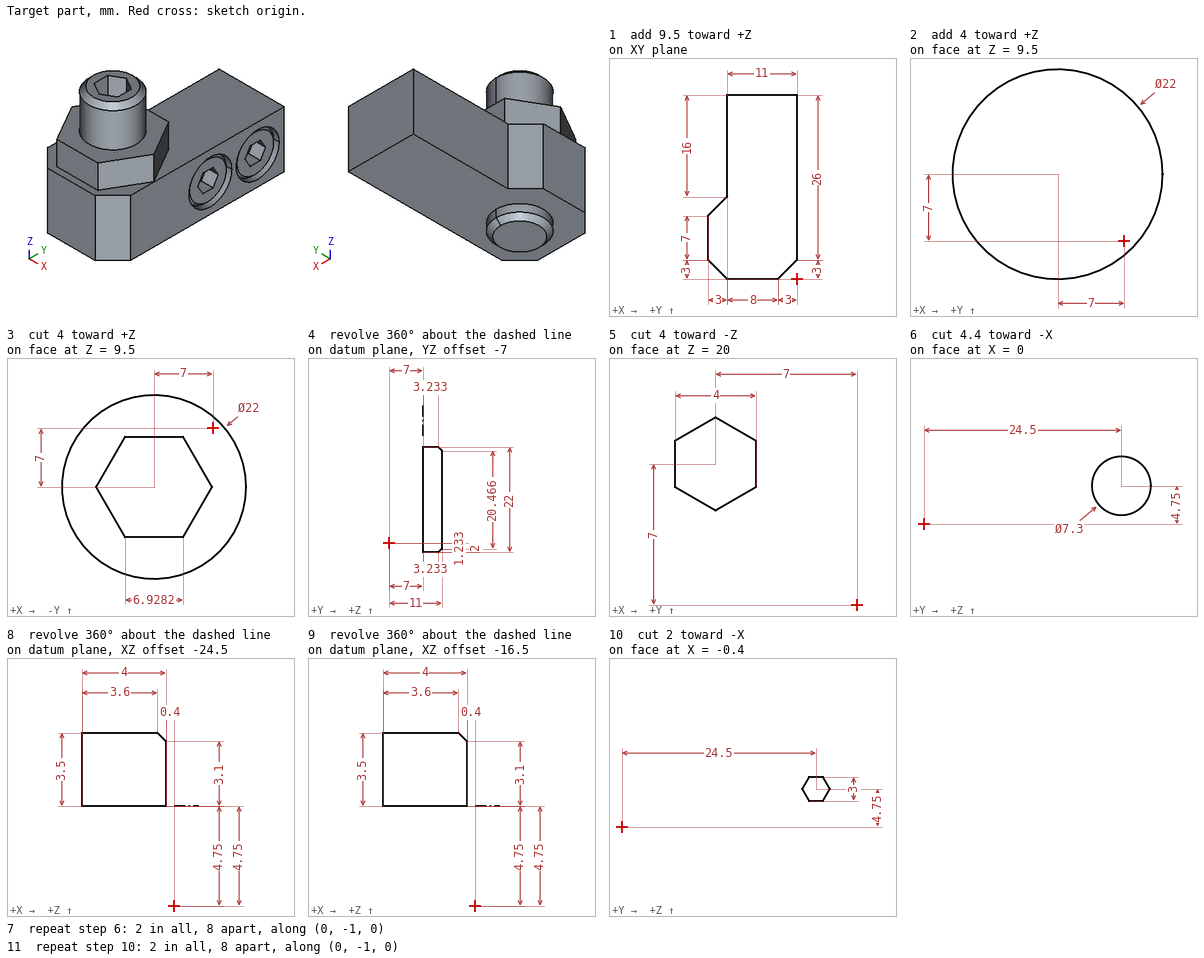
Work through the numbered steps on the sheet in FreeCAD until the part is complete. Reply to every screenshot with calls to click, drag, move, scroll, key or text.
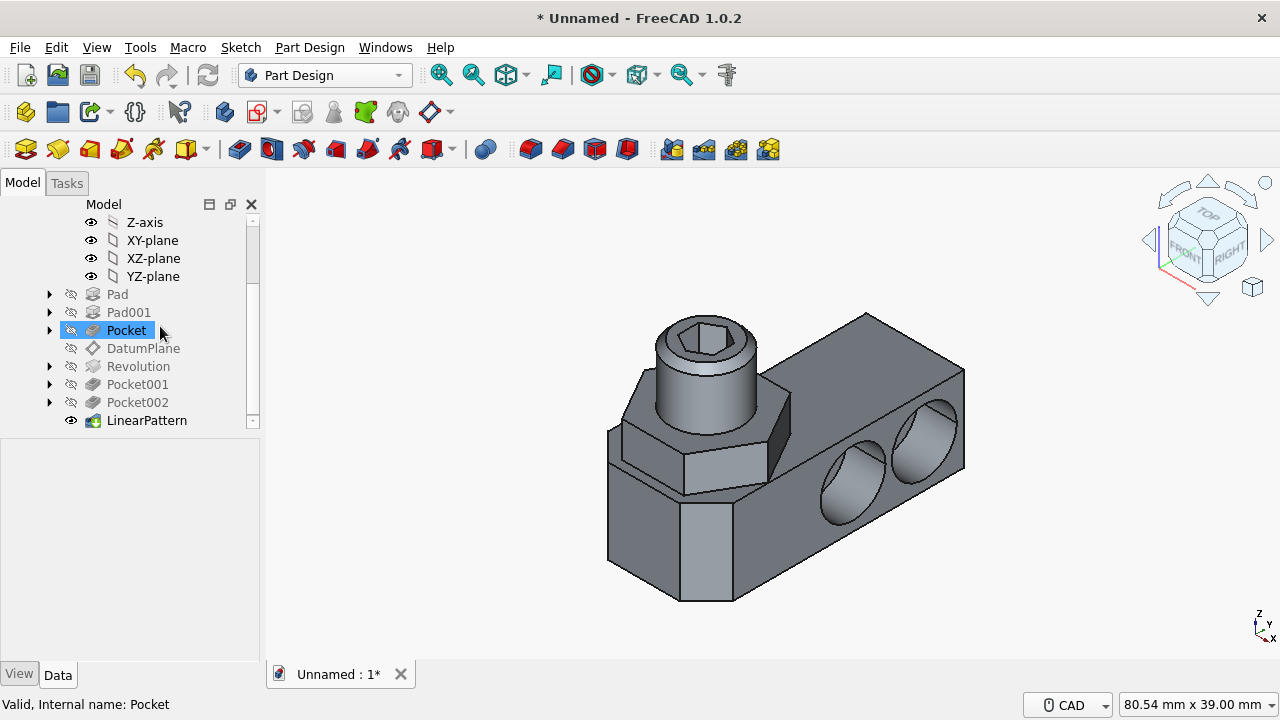
scroll(160, 326, up, 15)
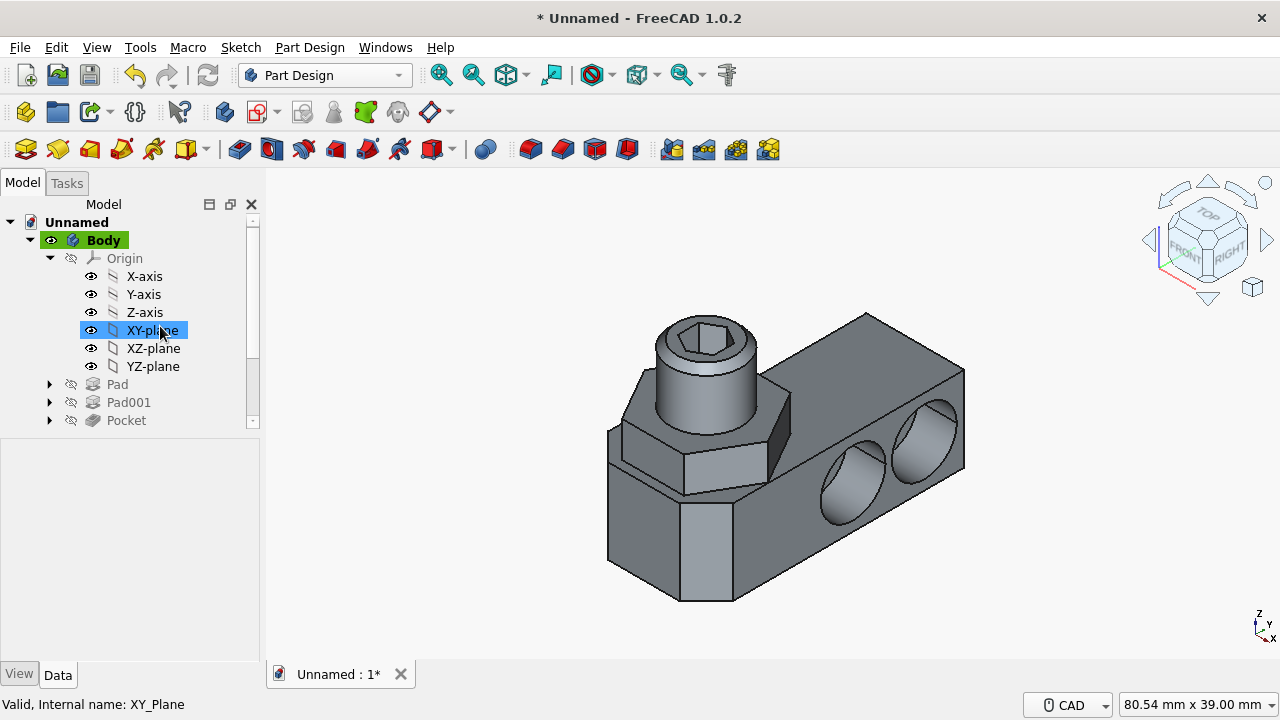
click(136, 348)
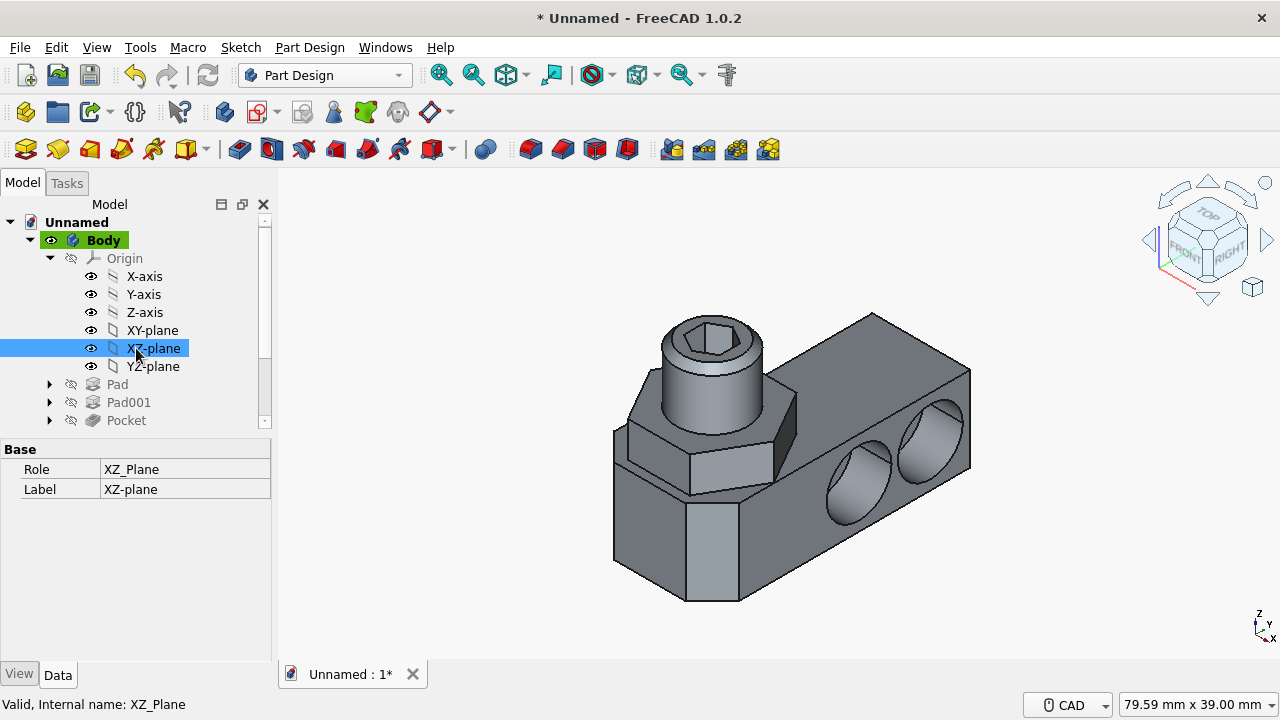
click(430, 112)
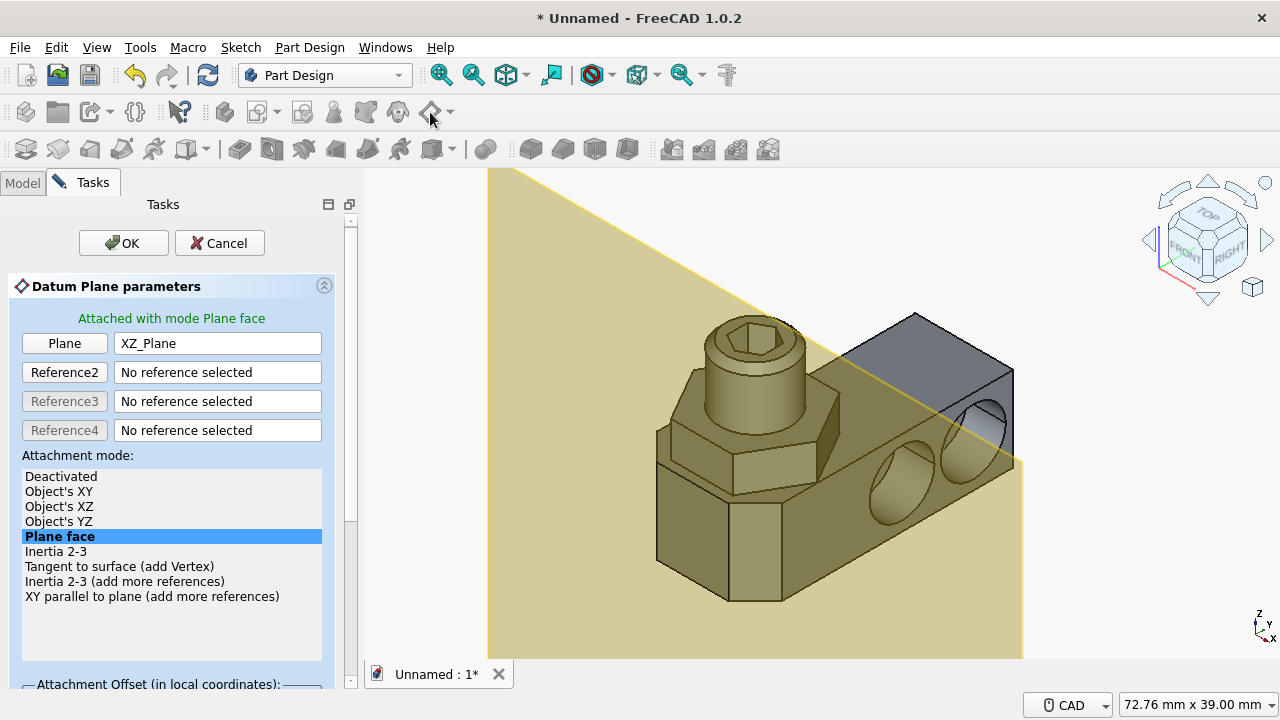
scroll(351, 451, down, 3)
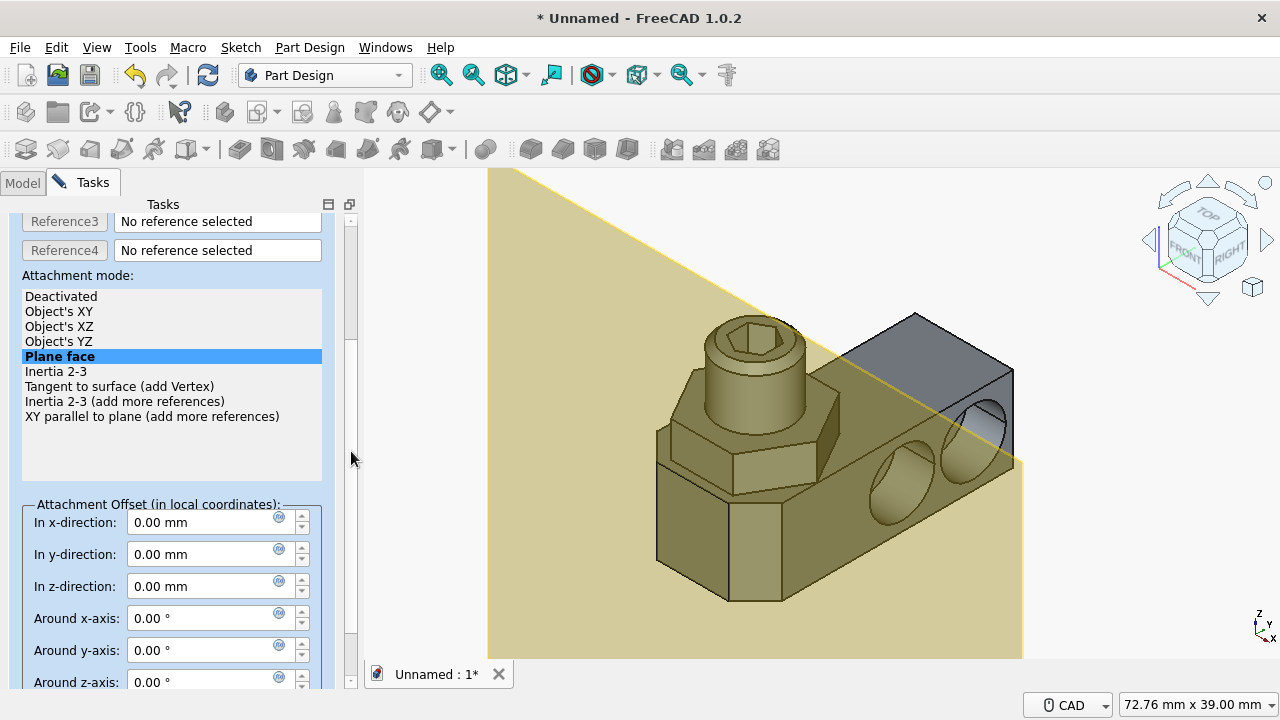
triple_click(210, 586)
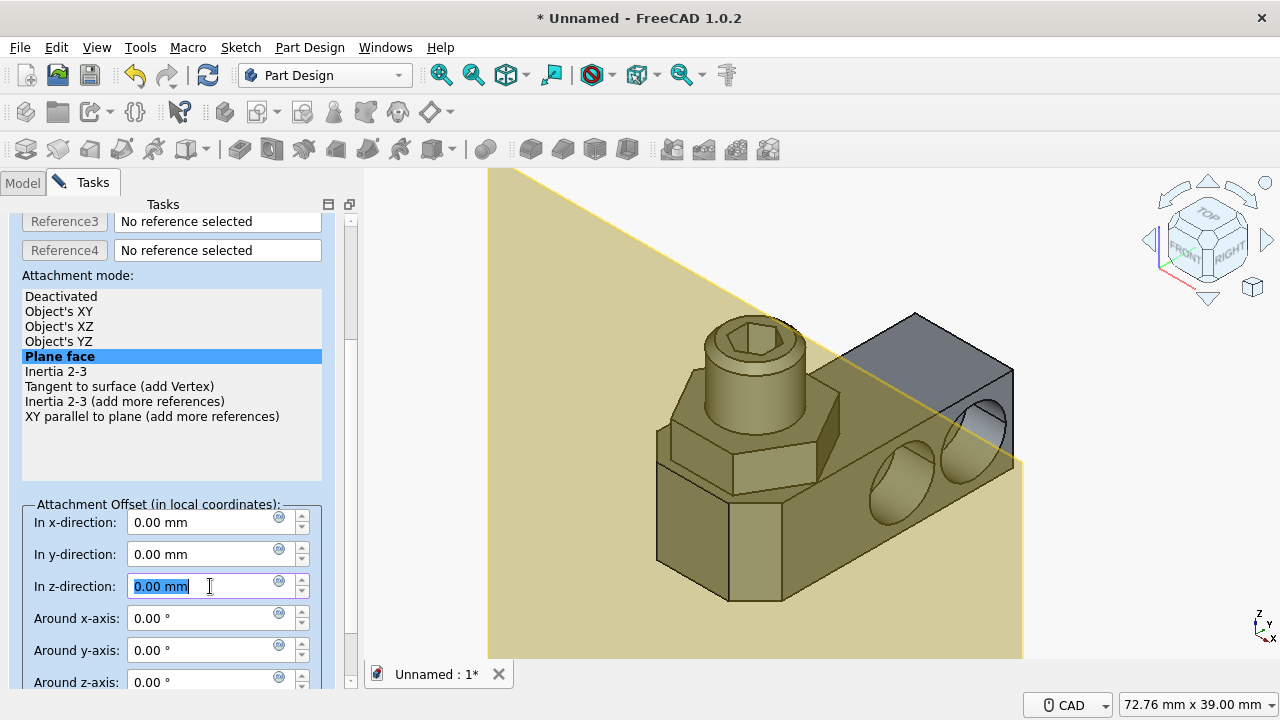
text(-24.5)
key(Tab)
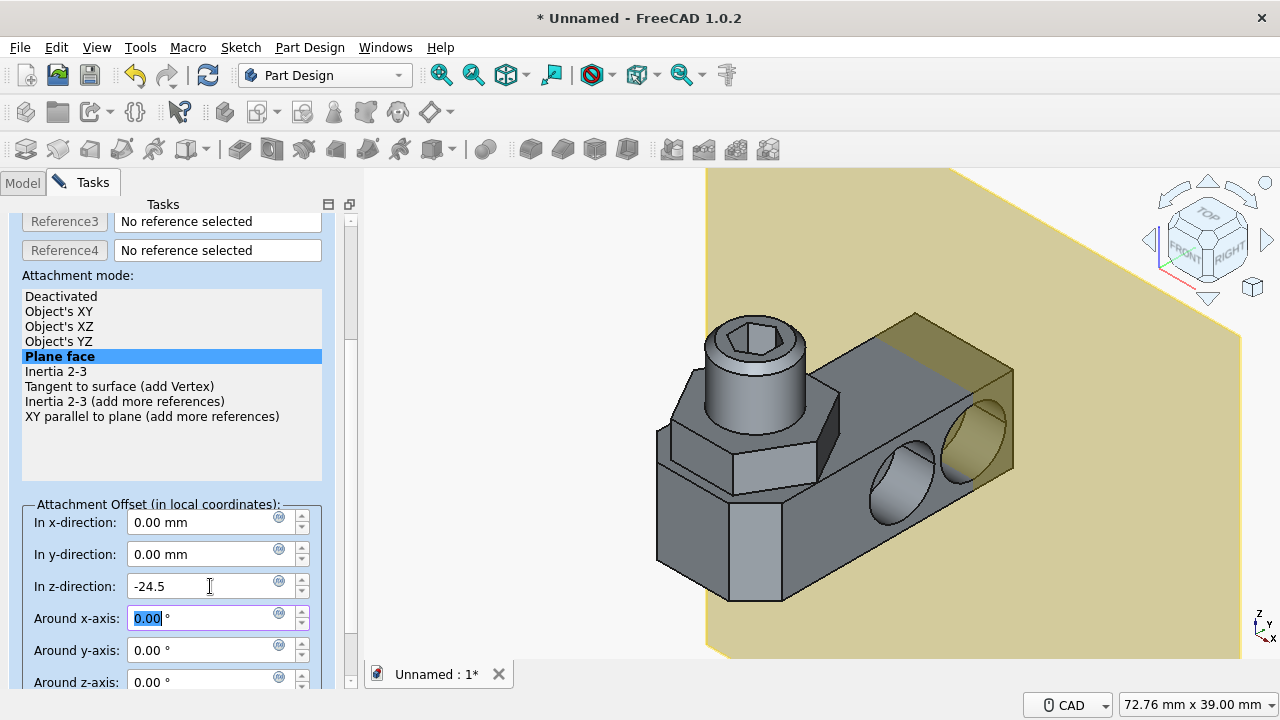
scroll(351, 451, up, 4)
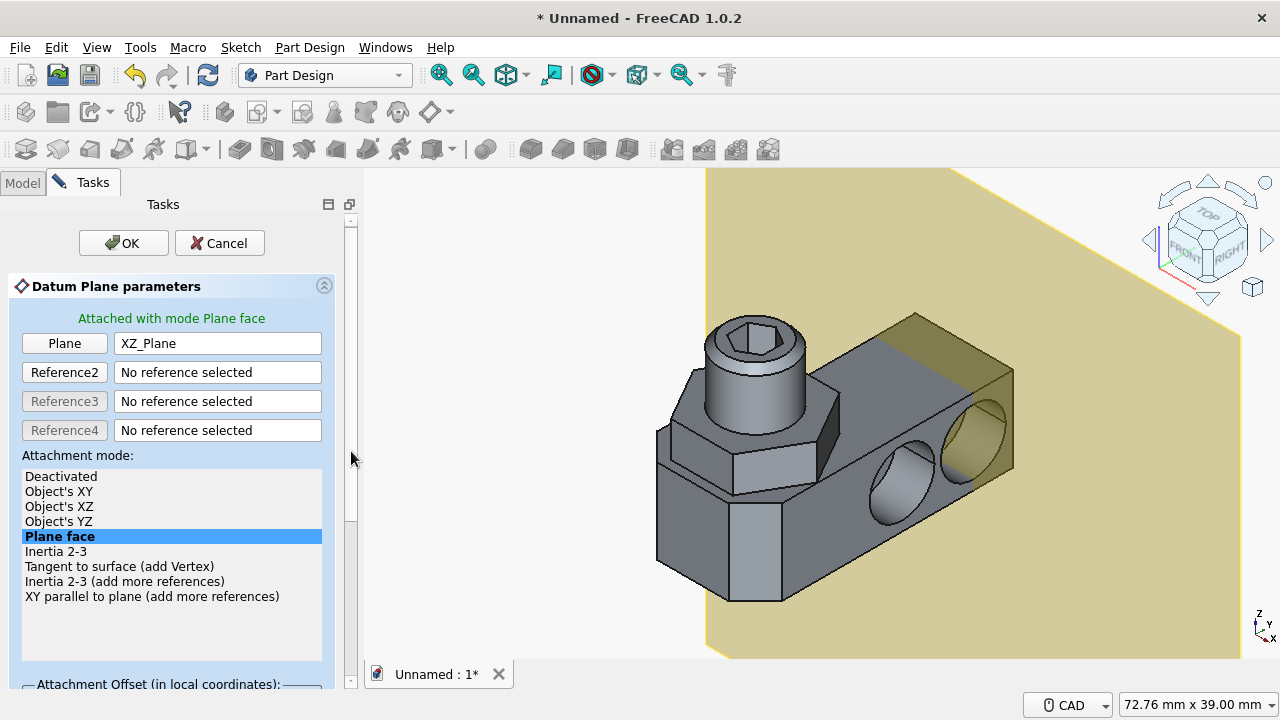
click(124, 243)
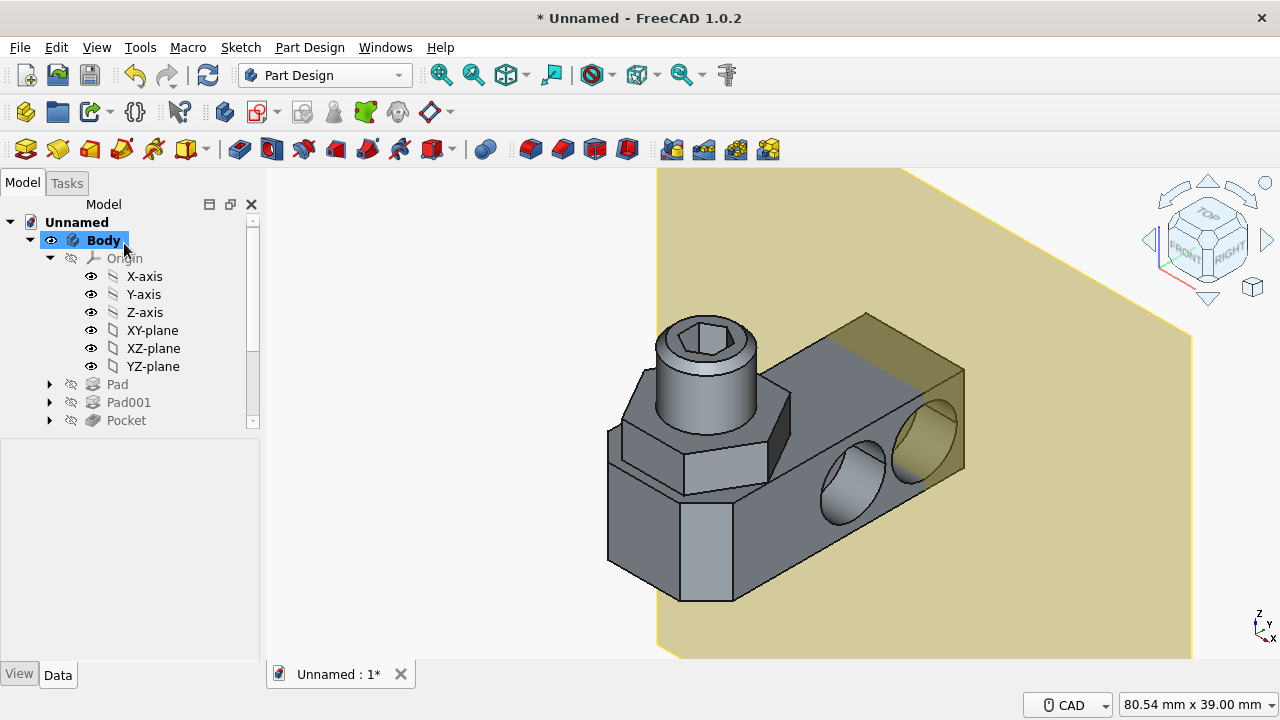
scroll(100, 326, down, 3)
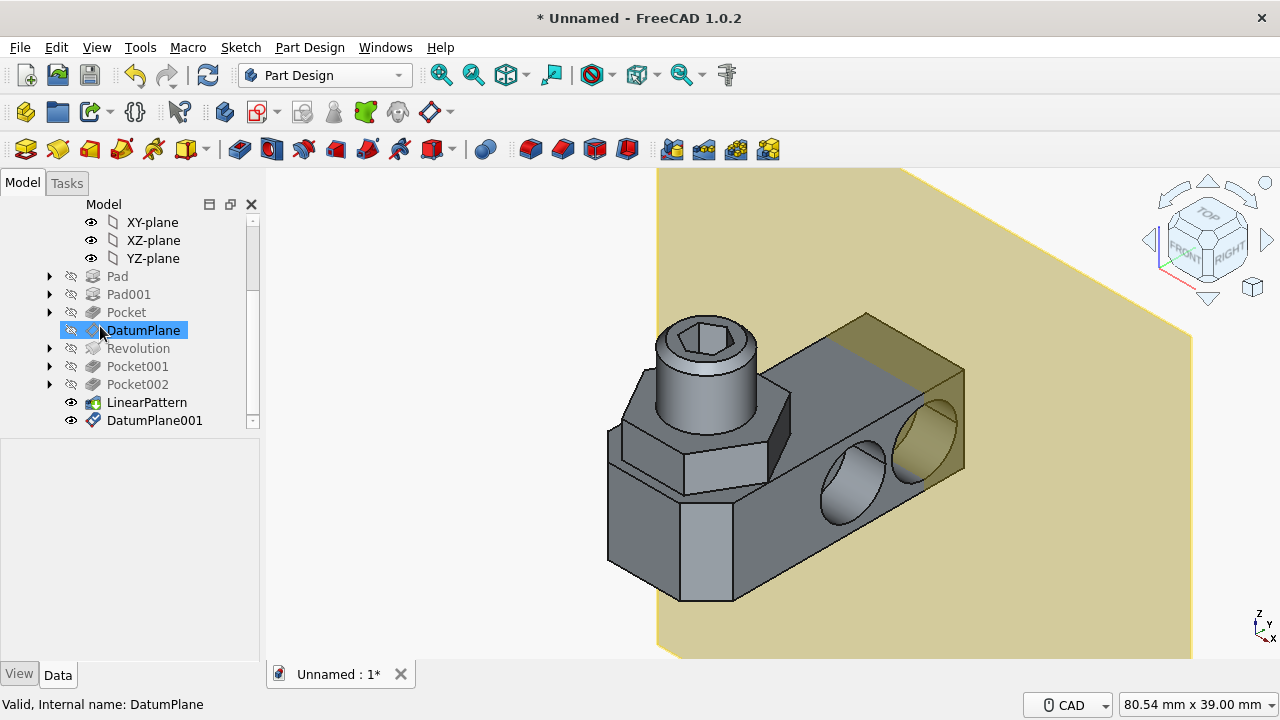
click(116, 420)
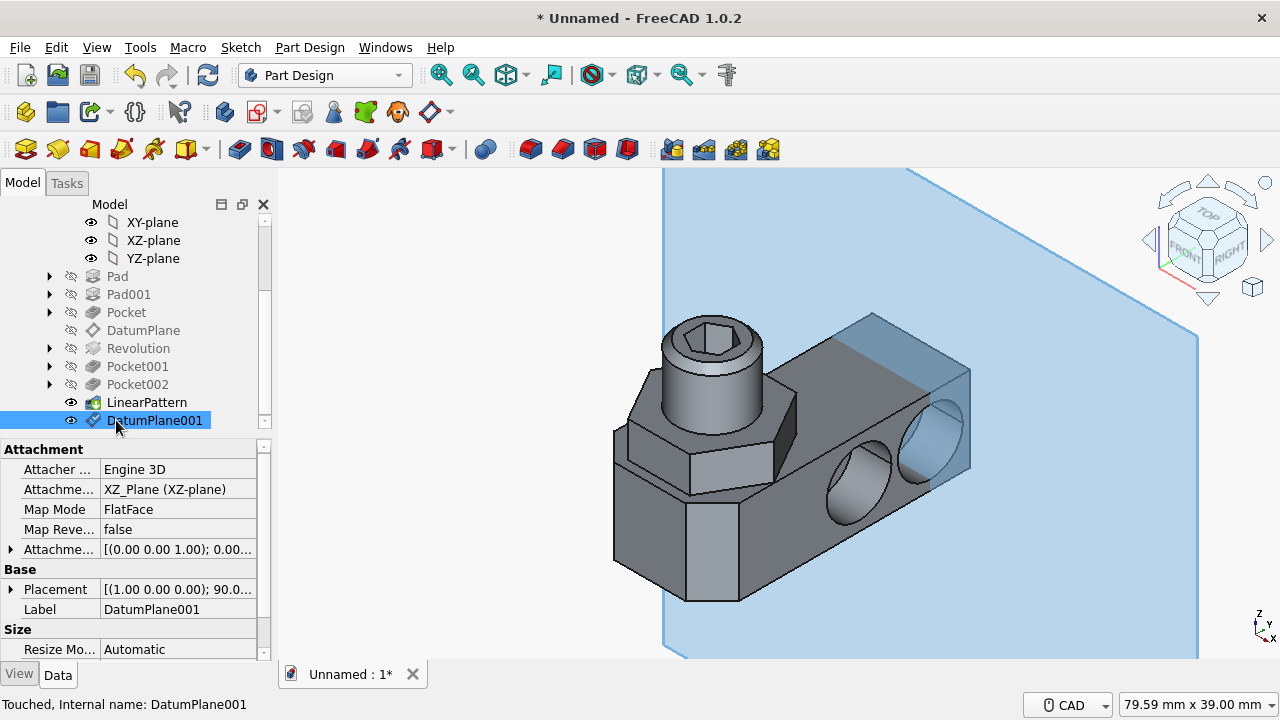
click(258, 112)